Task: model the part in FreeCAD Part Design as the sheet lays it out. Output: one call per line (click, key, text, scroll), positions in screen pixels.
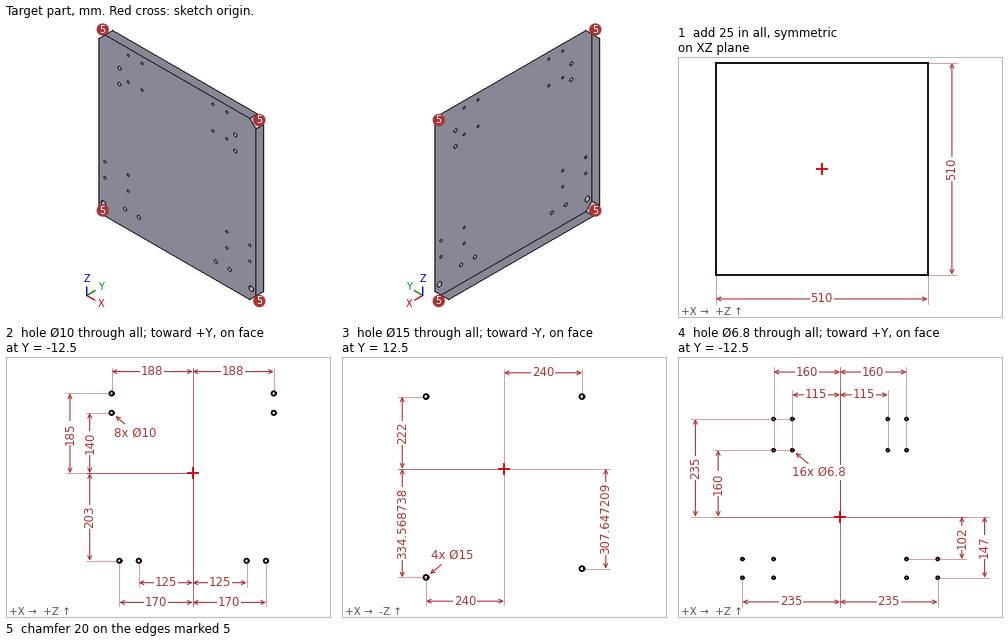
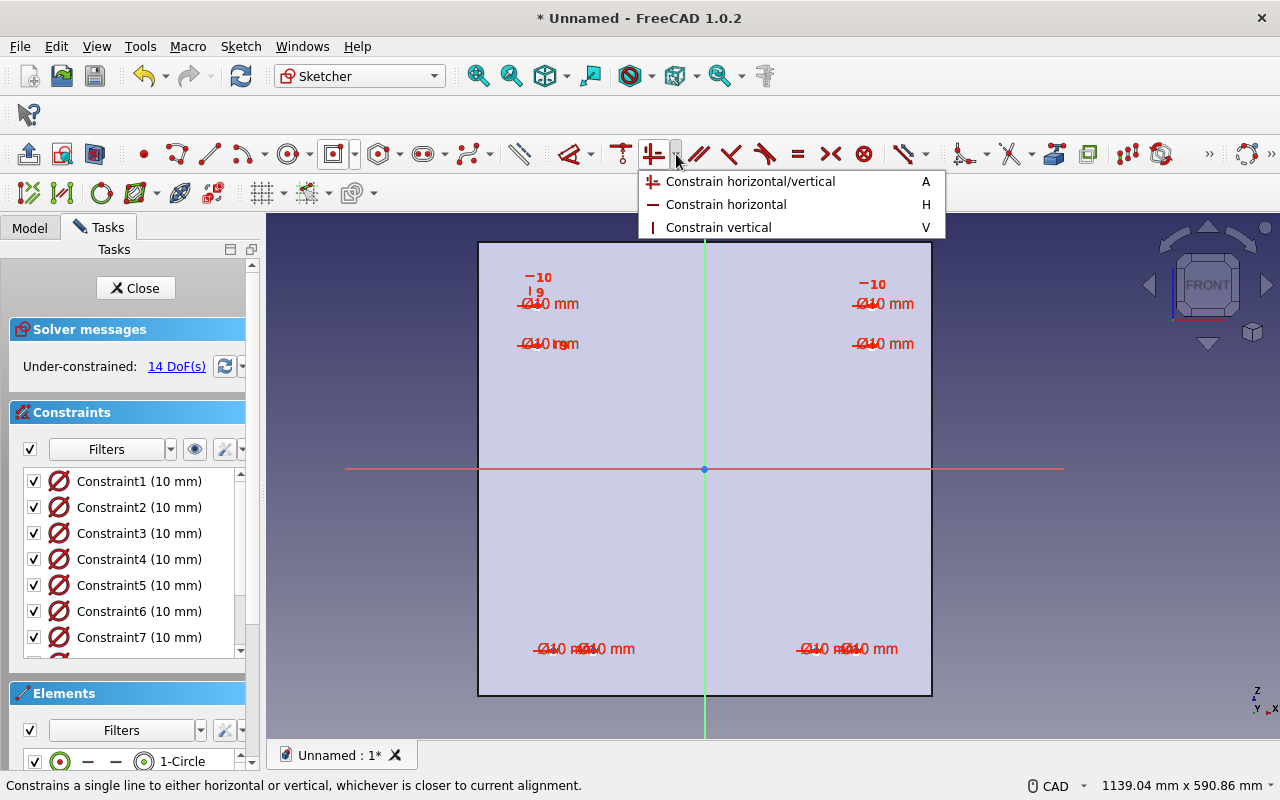
click(792, 228)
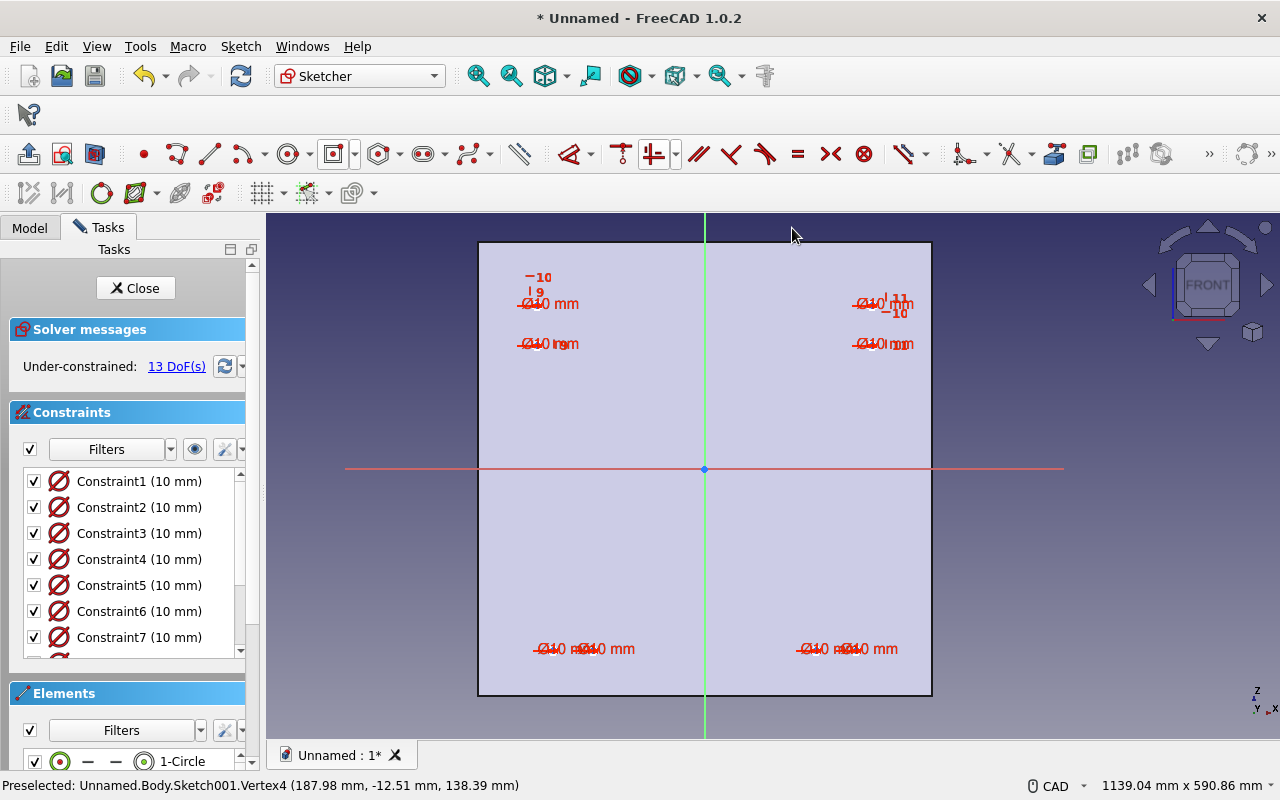
click(537, 346)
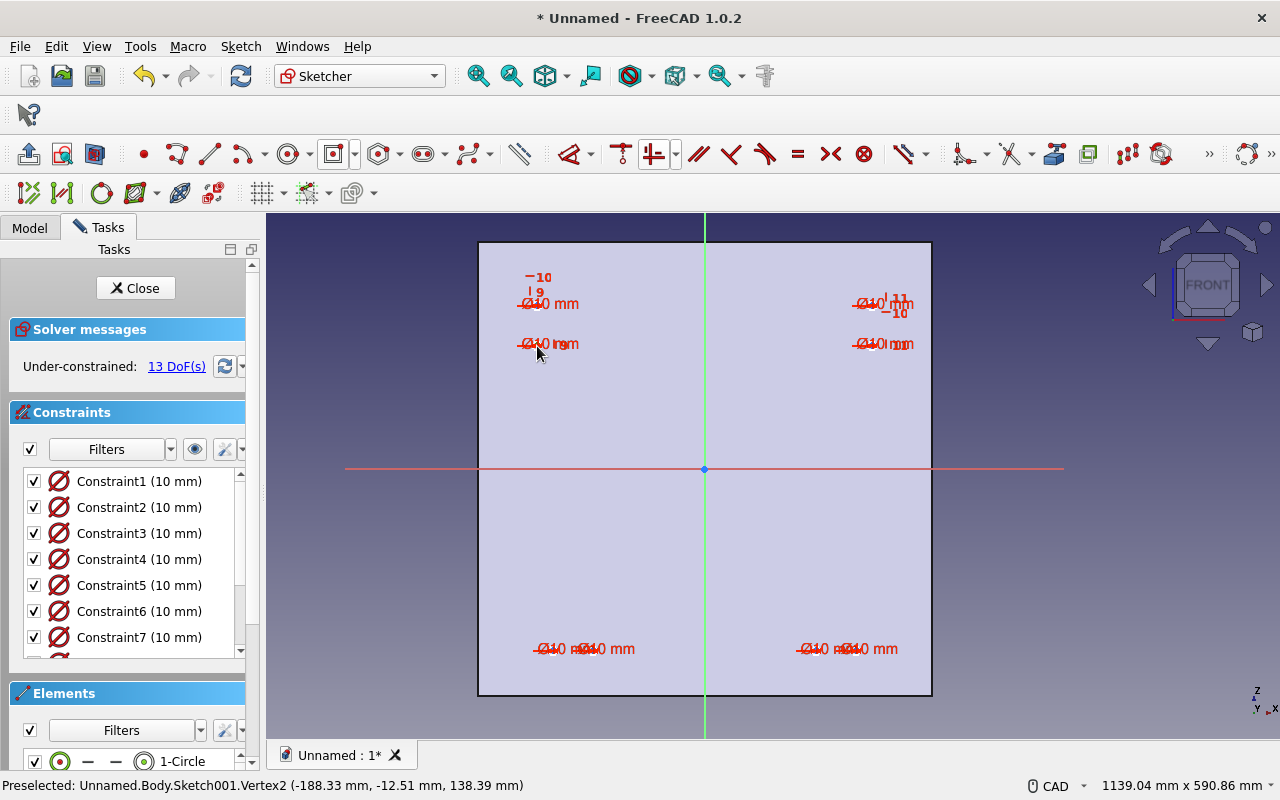
click(872, 346)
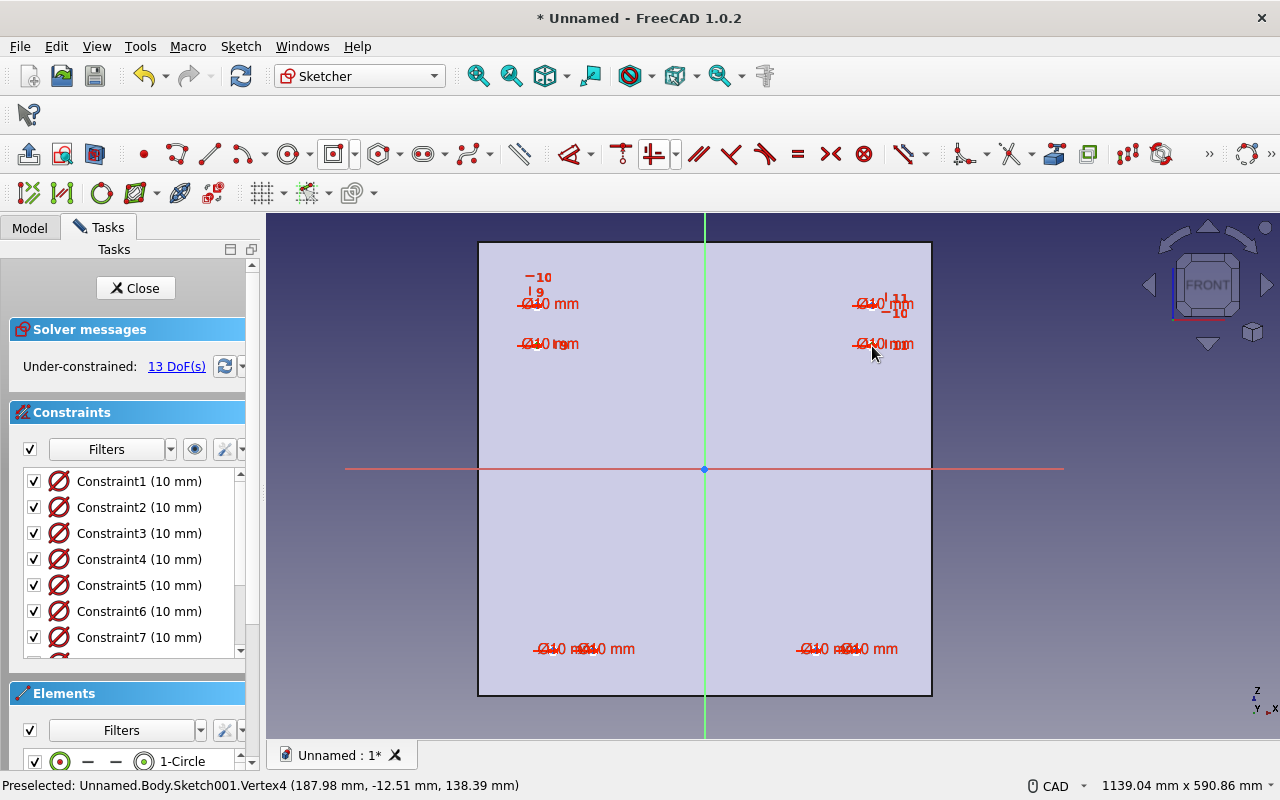
click(676, 154)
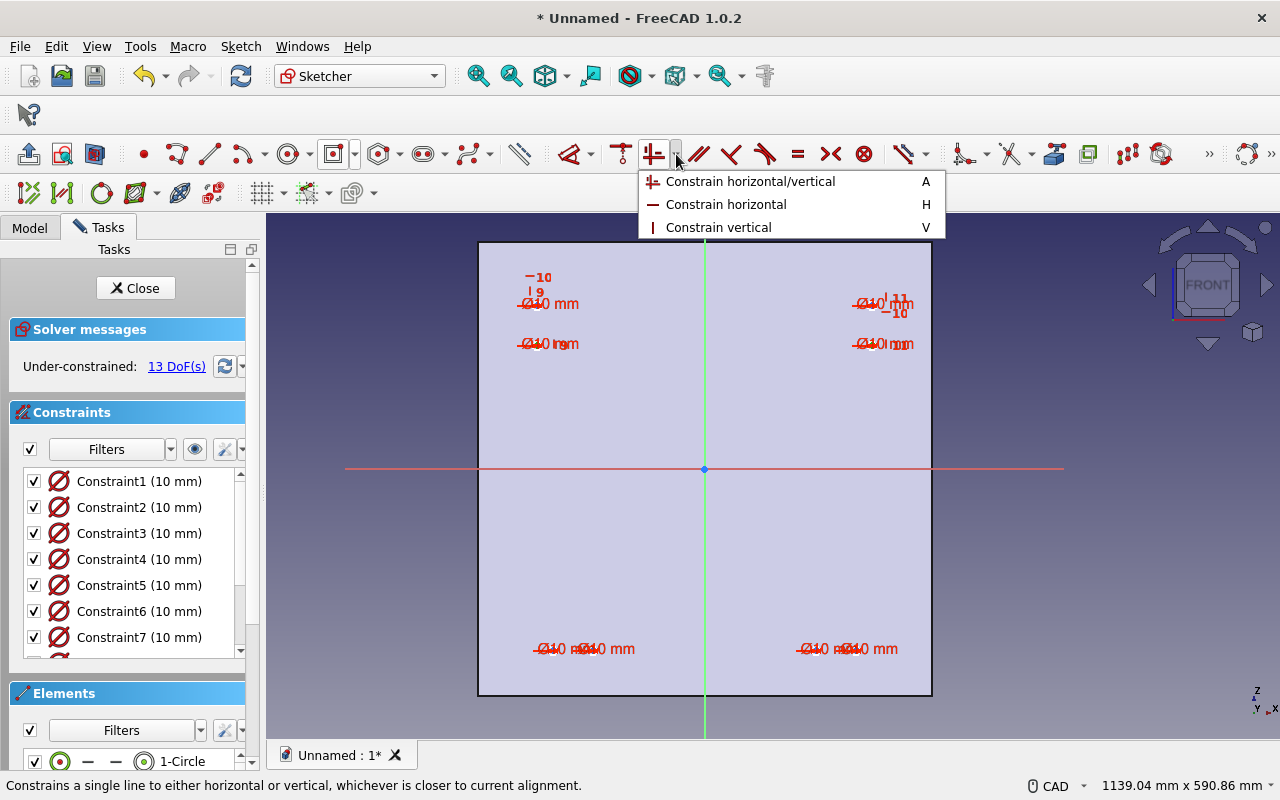
click(792, 204)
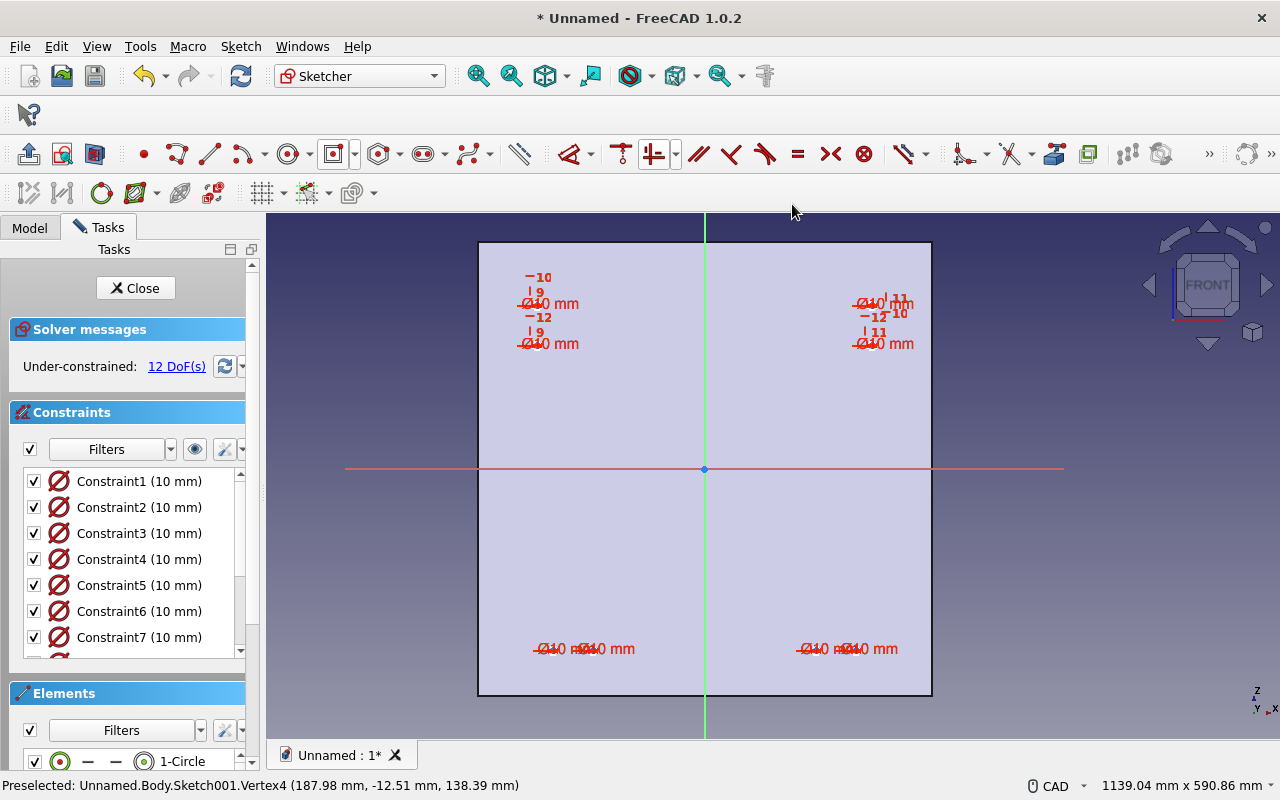
click(553, 651)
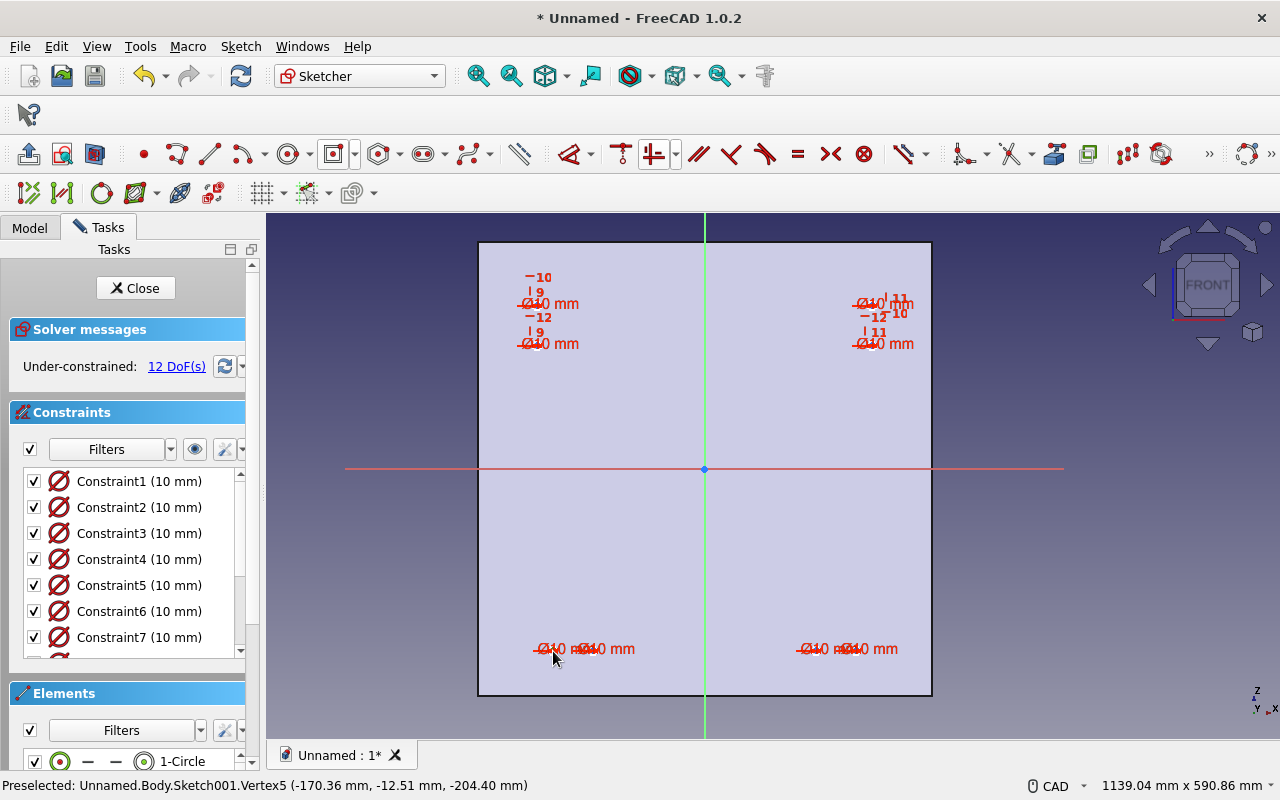
click(593, 651)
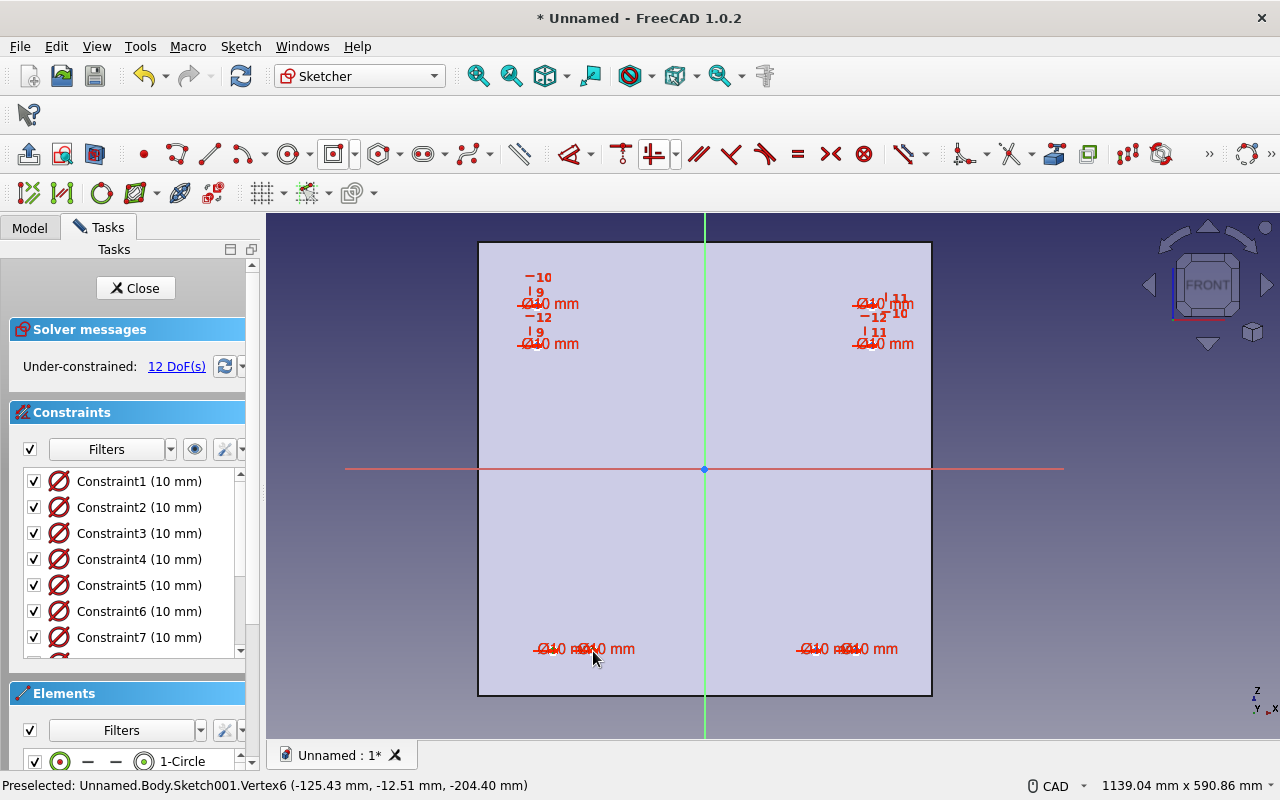
click(676, 154)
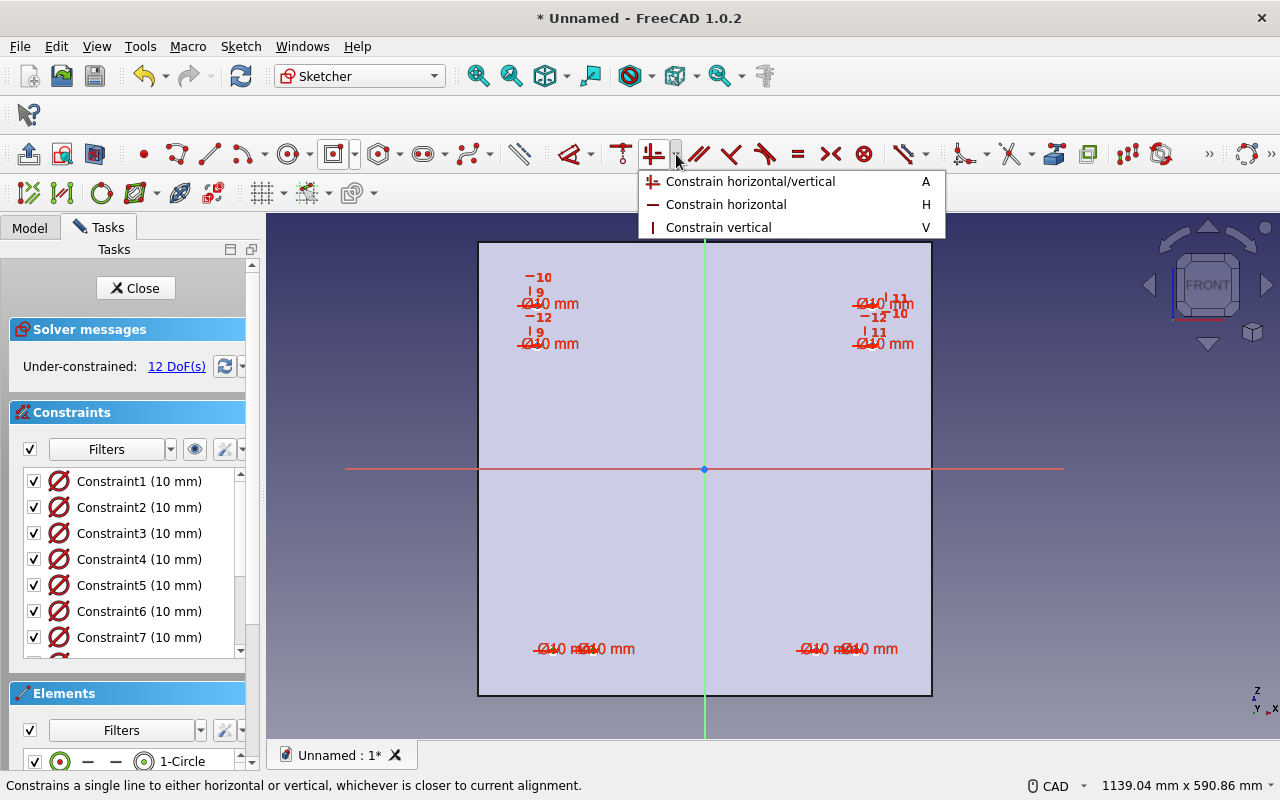
click(792, 204)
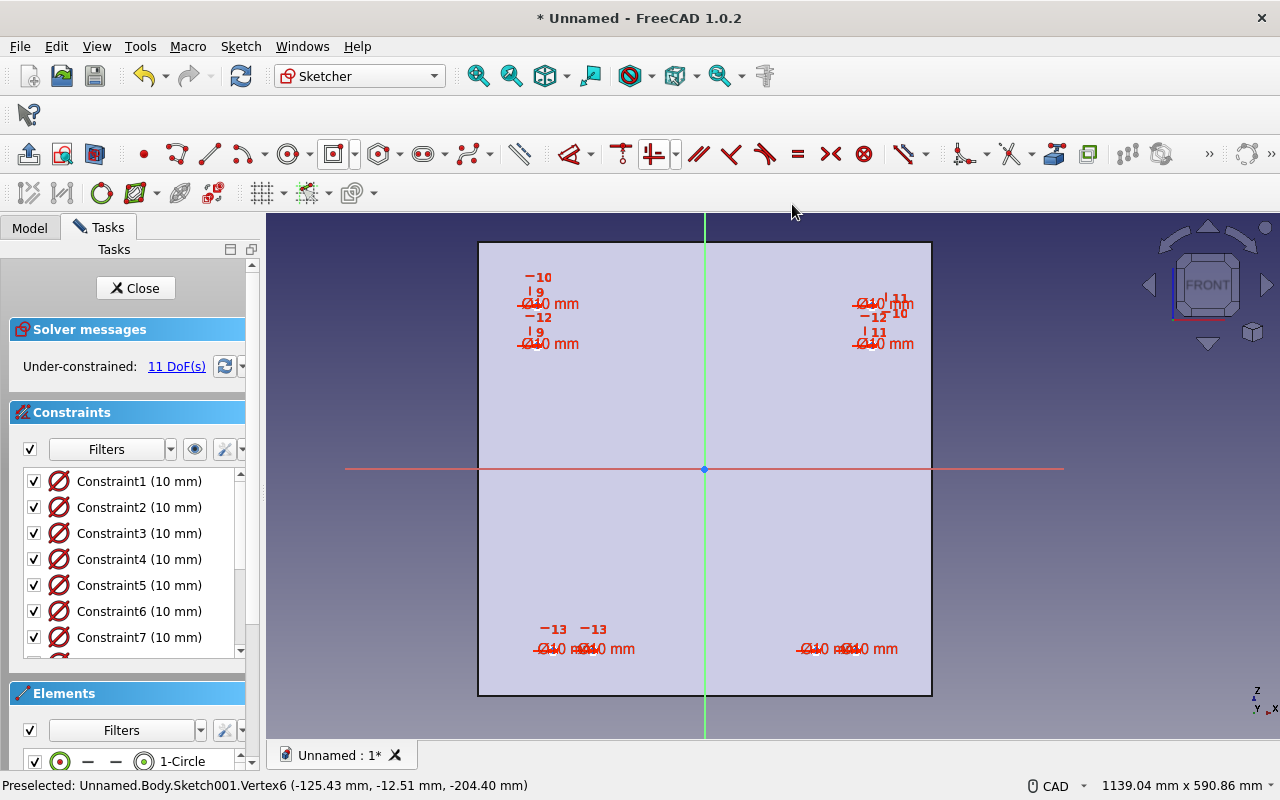
click(593, 651)